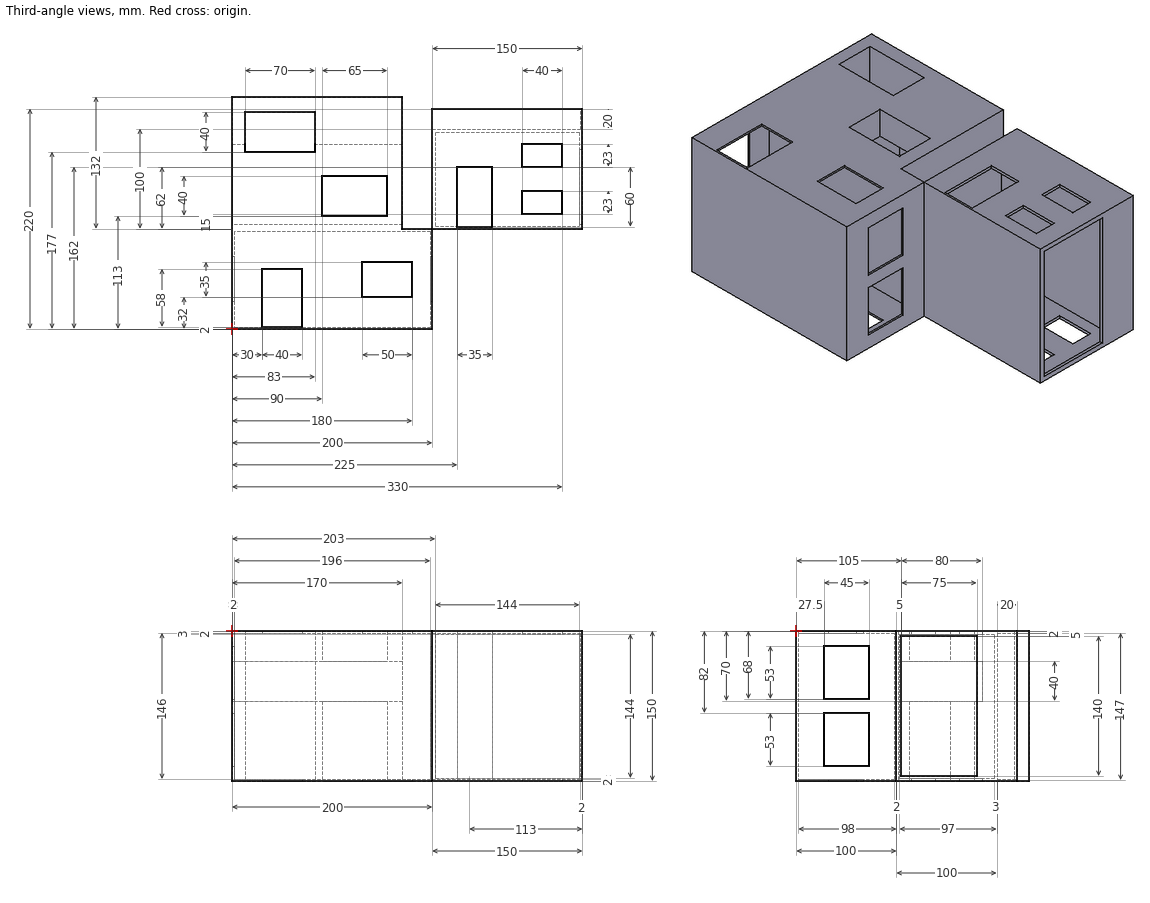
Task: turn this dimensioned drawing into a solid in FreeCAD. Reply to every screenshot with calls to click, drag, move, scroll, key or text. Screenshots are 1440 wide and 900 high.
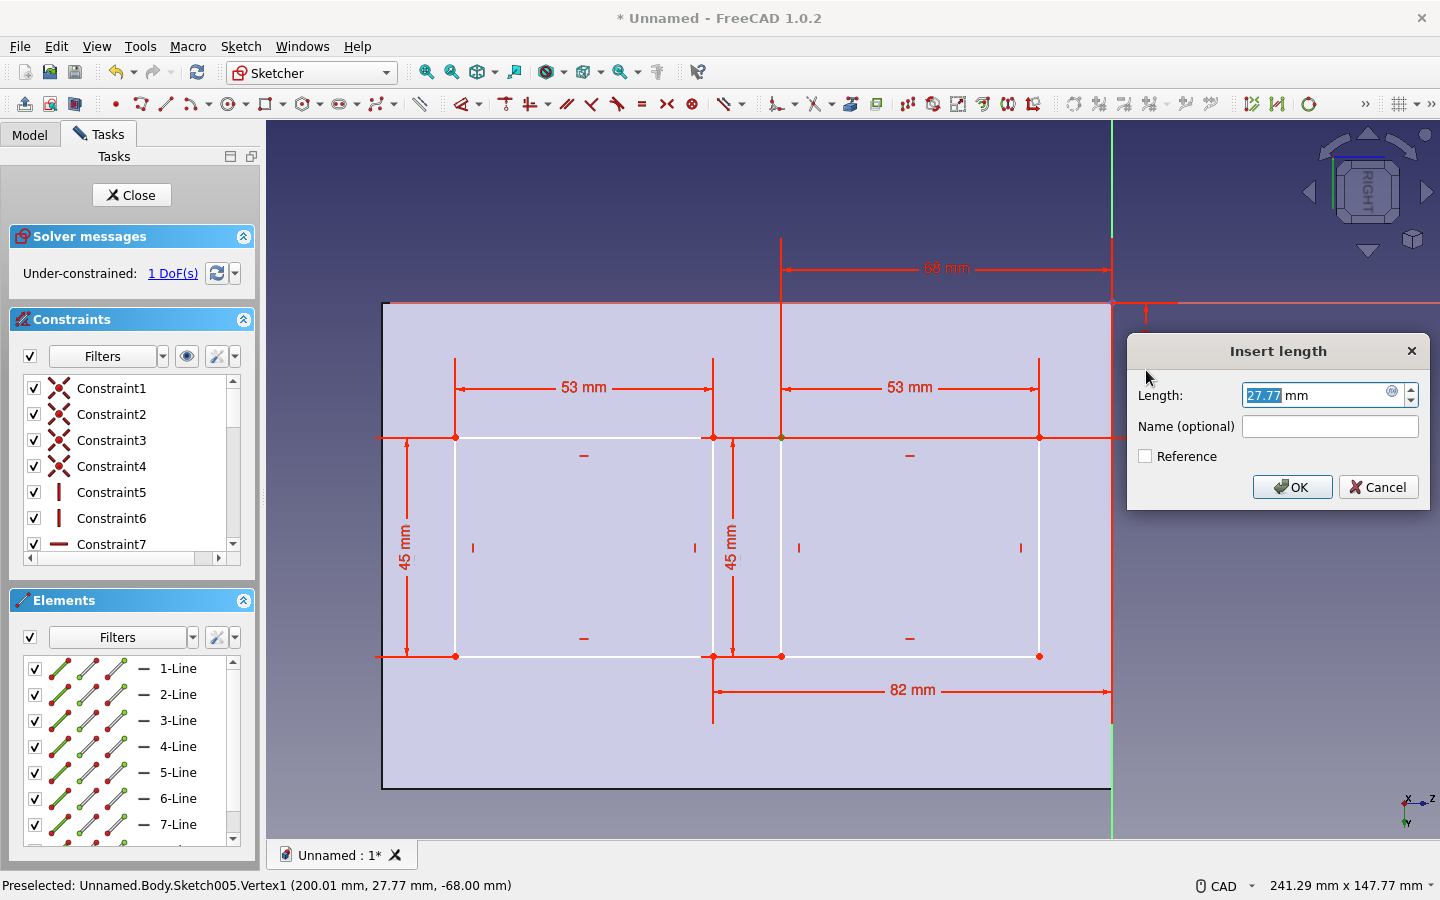
text(27.5)
key(Return)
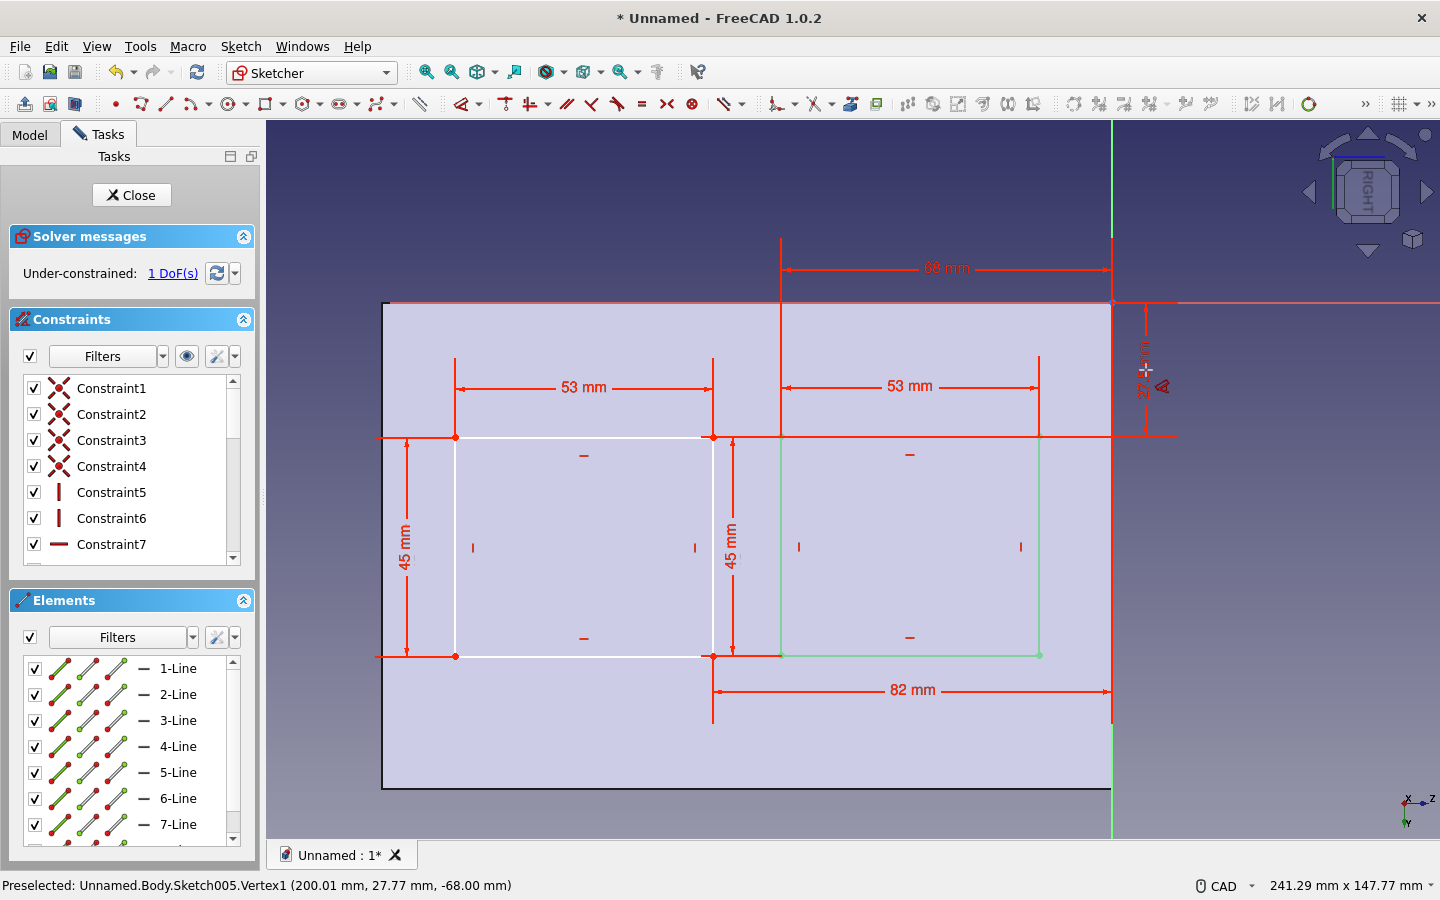
click(455, 438)
click(1146, 339)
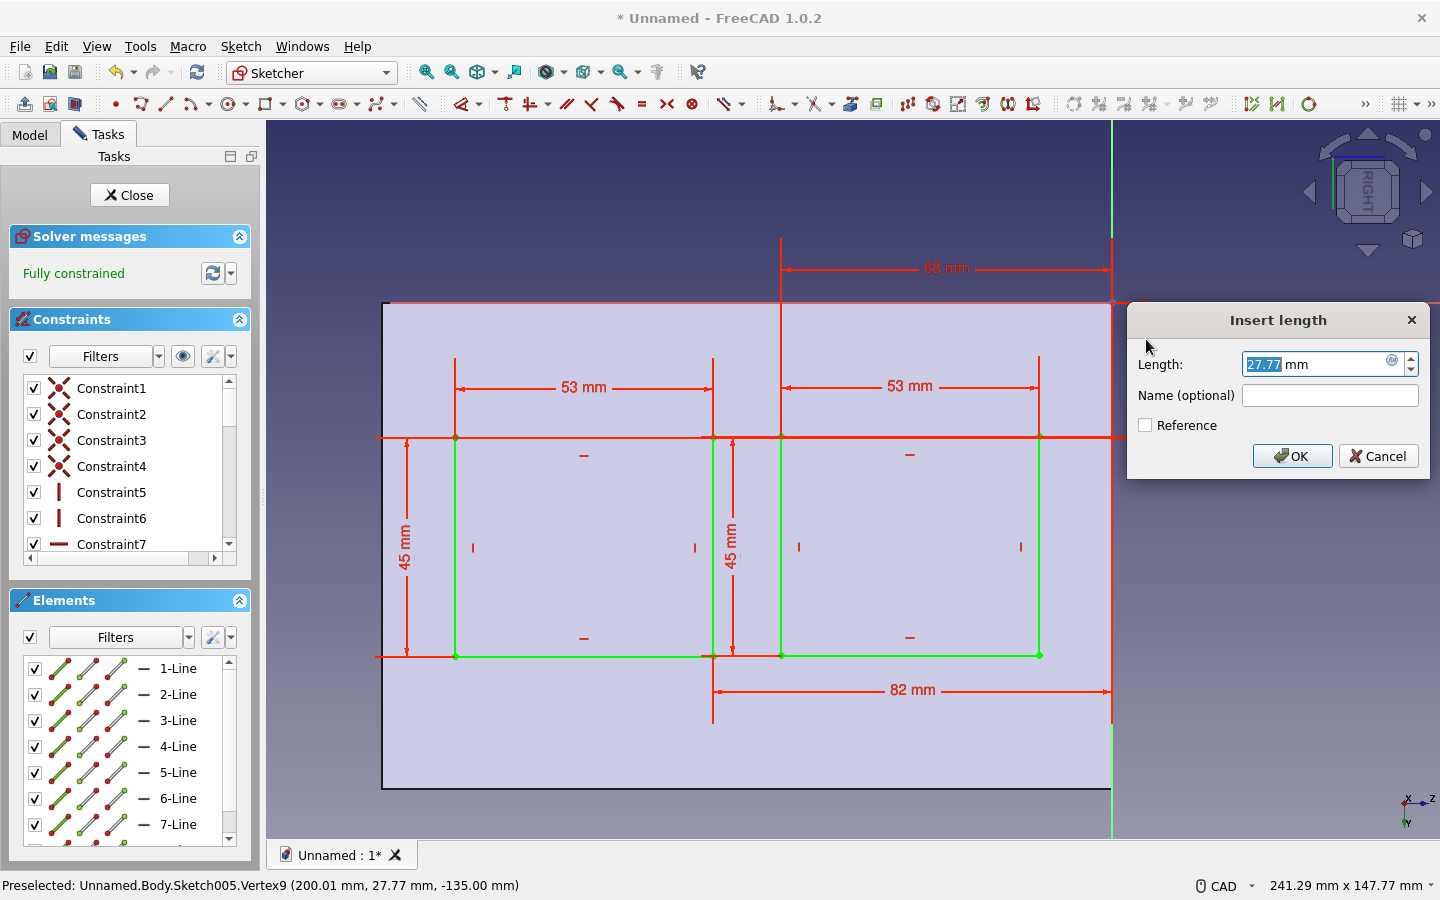
text(27.5)
key(Return)
key(Escape)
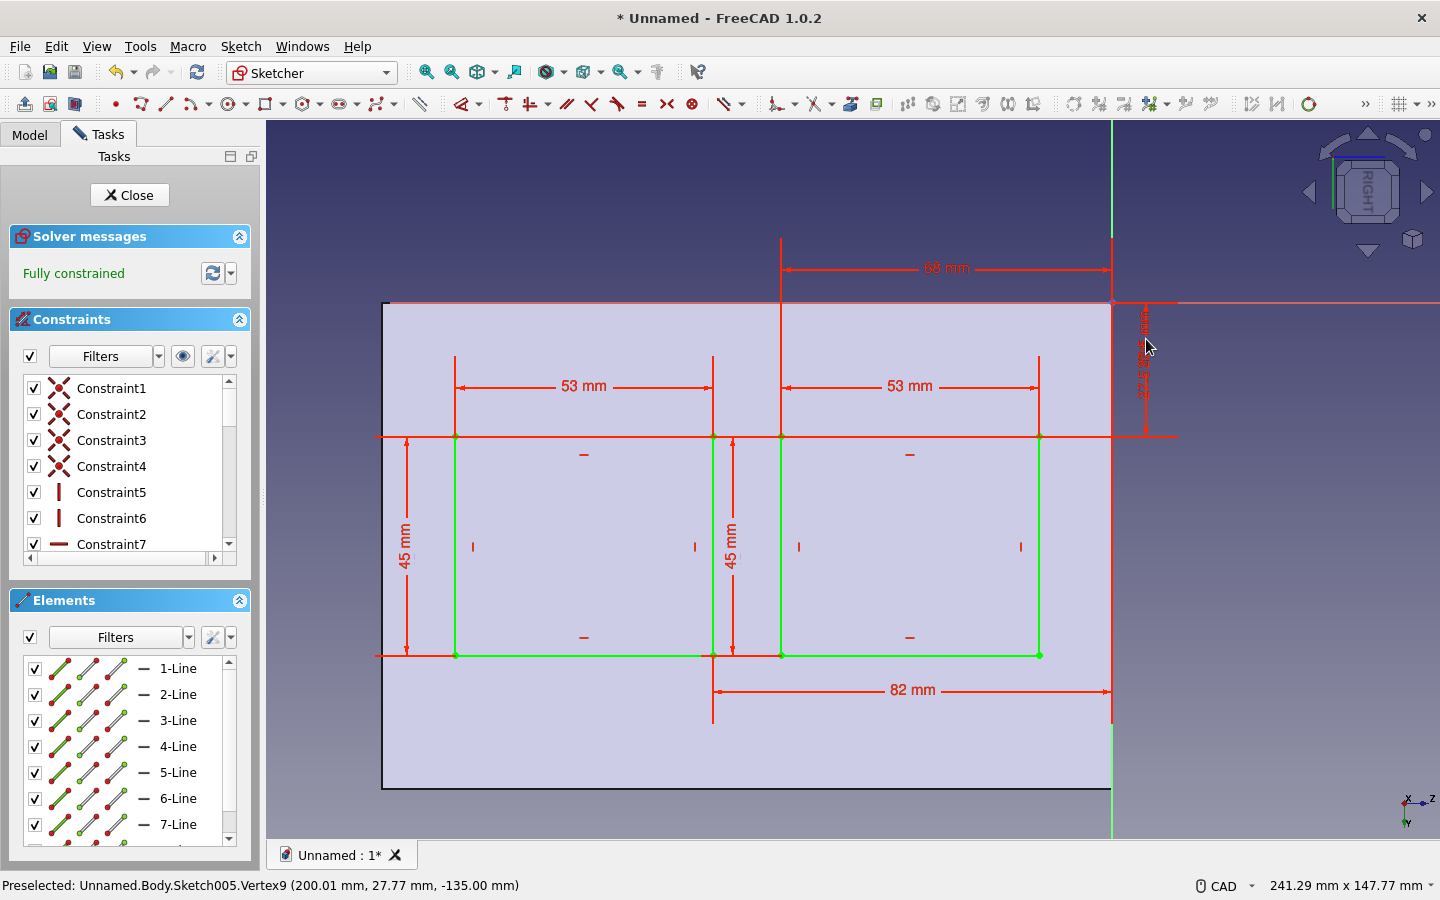
click(130, 195)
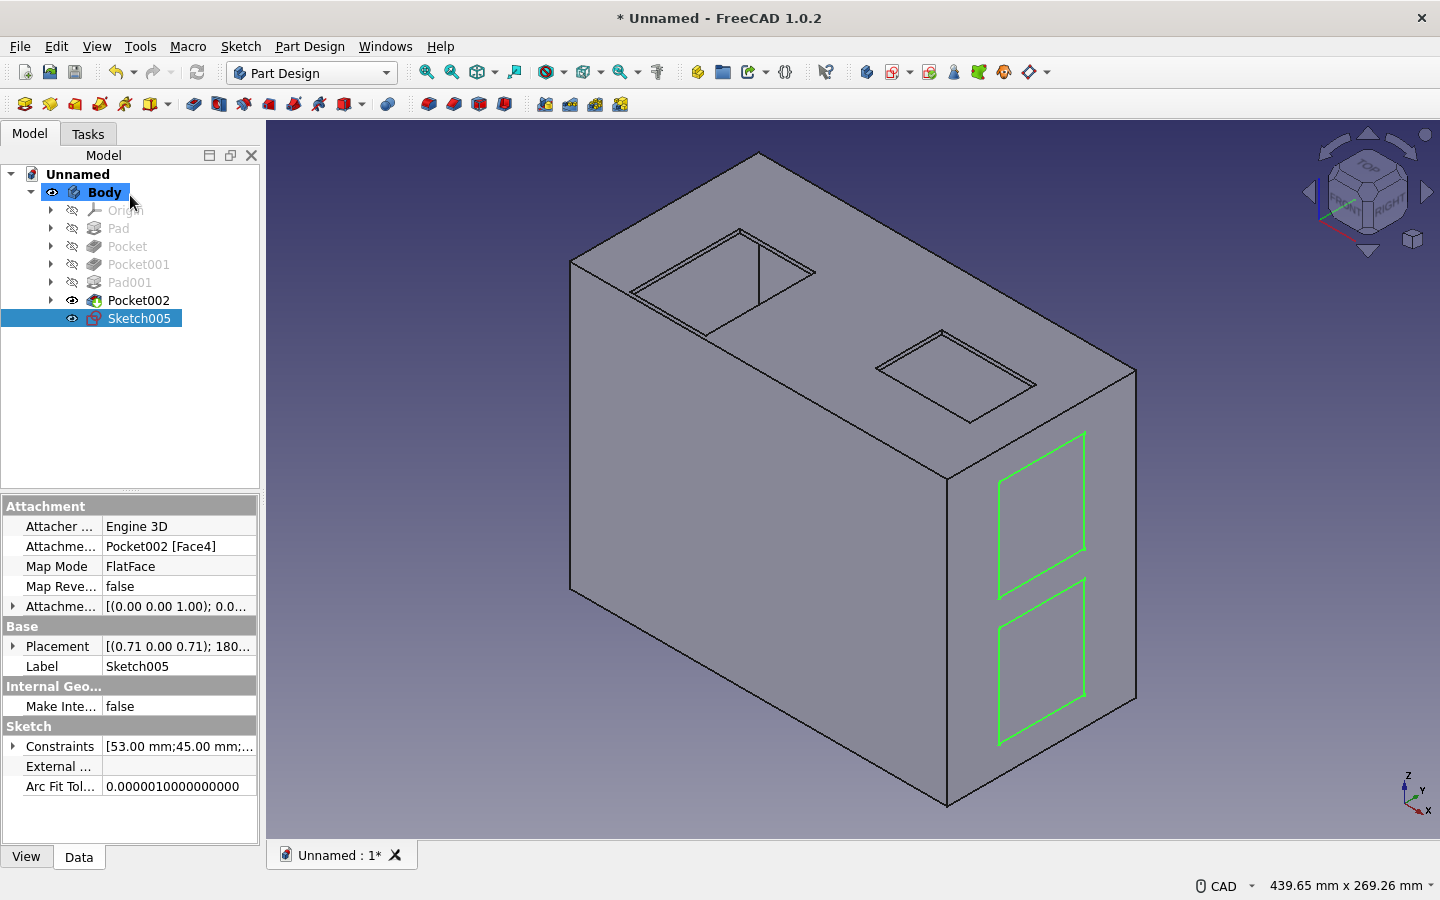
click(194, 104)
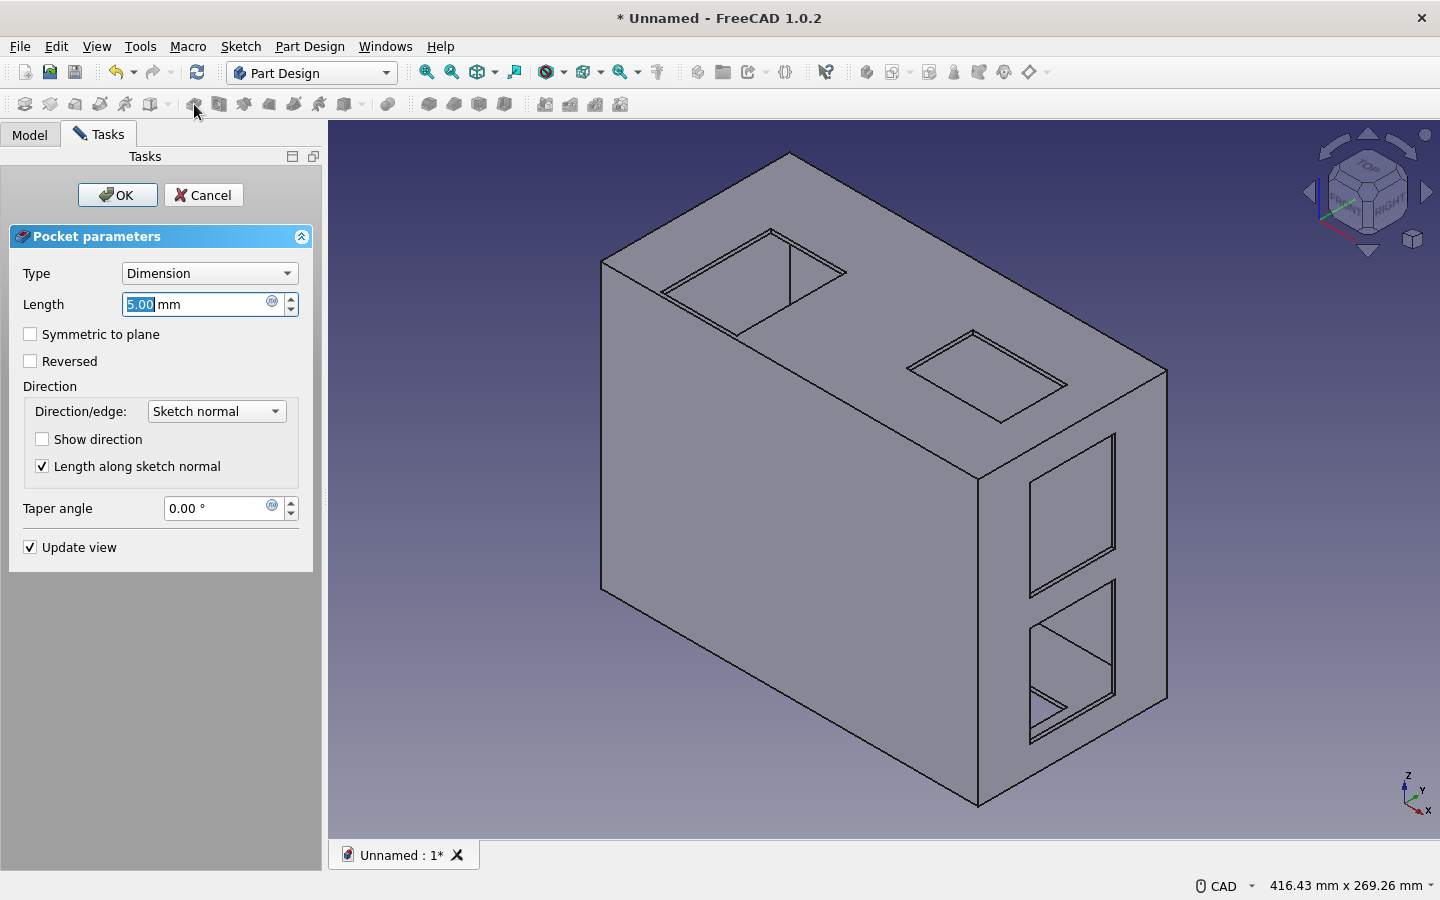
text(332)
key(Tab)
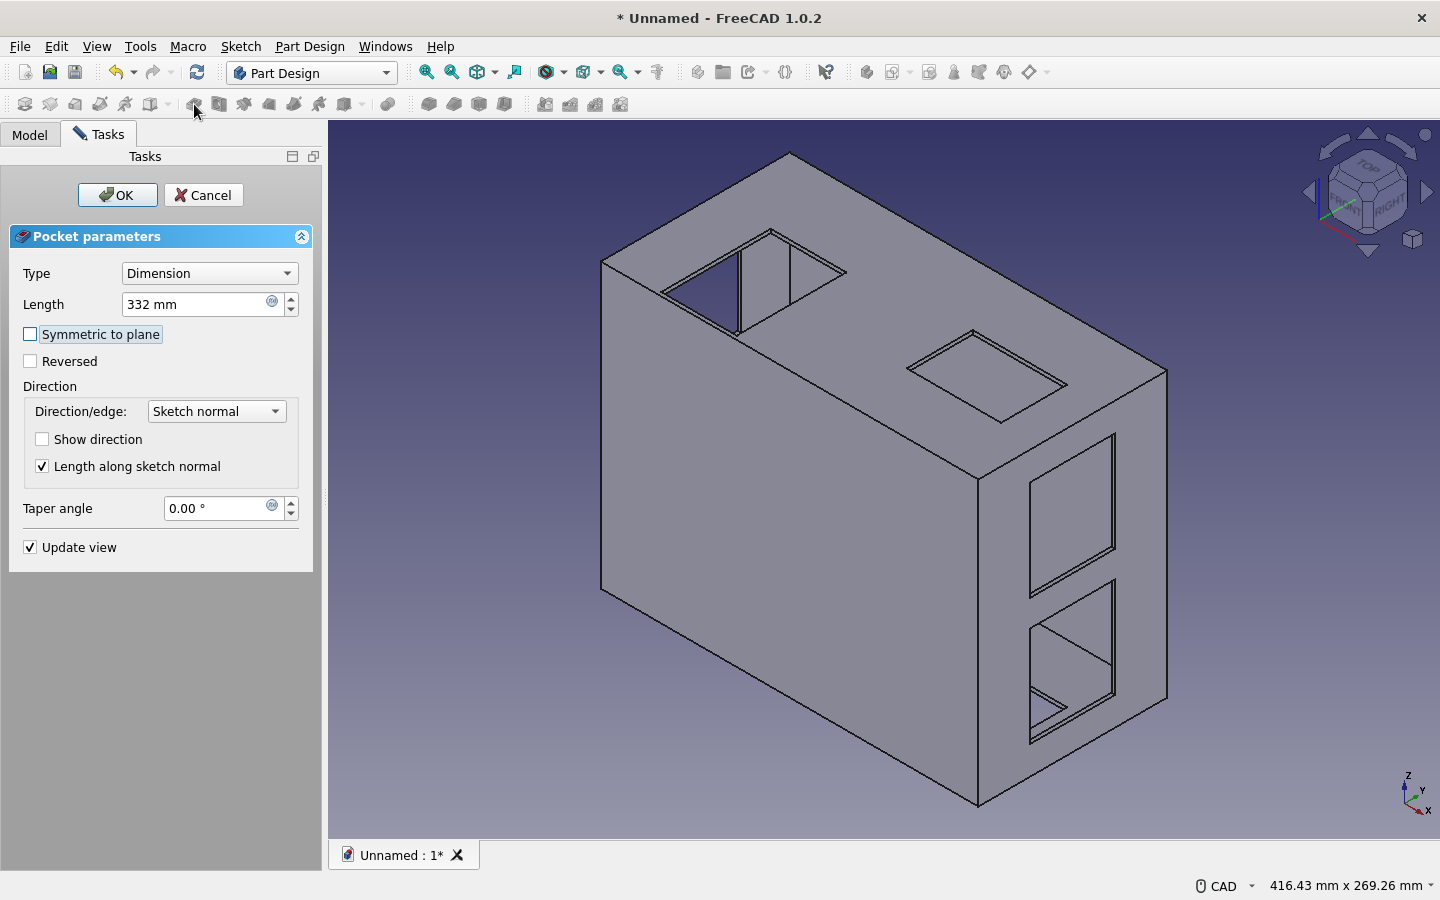
click(118, 195)